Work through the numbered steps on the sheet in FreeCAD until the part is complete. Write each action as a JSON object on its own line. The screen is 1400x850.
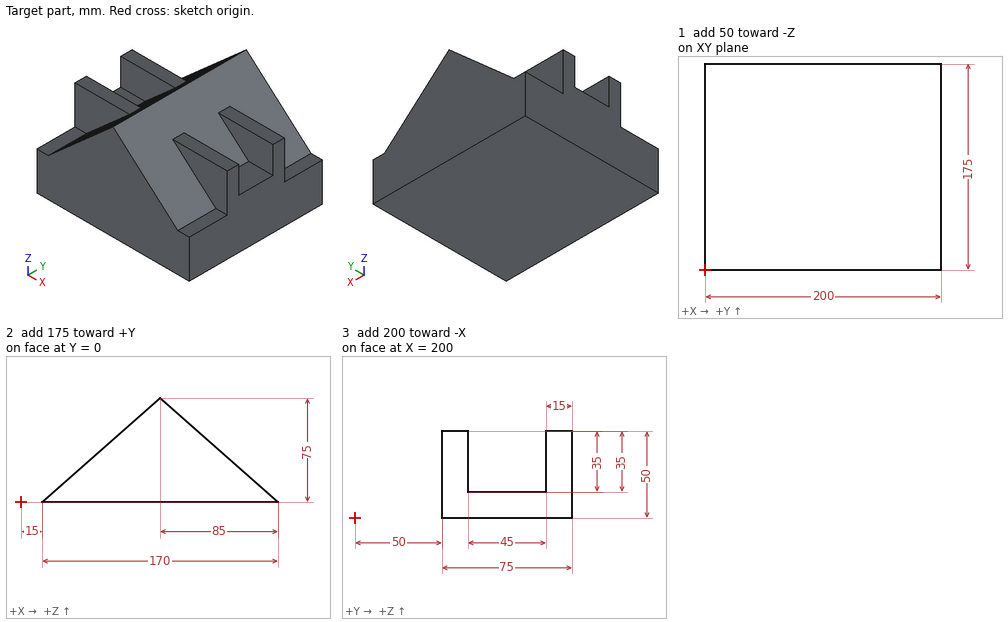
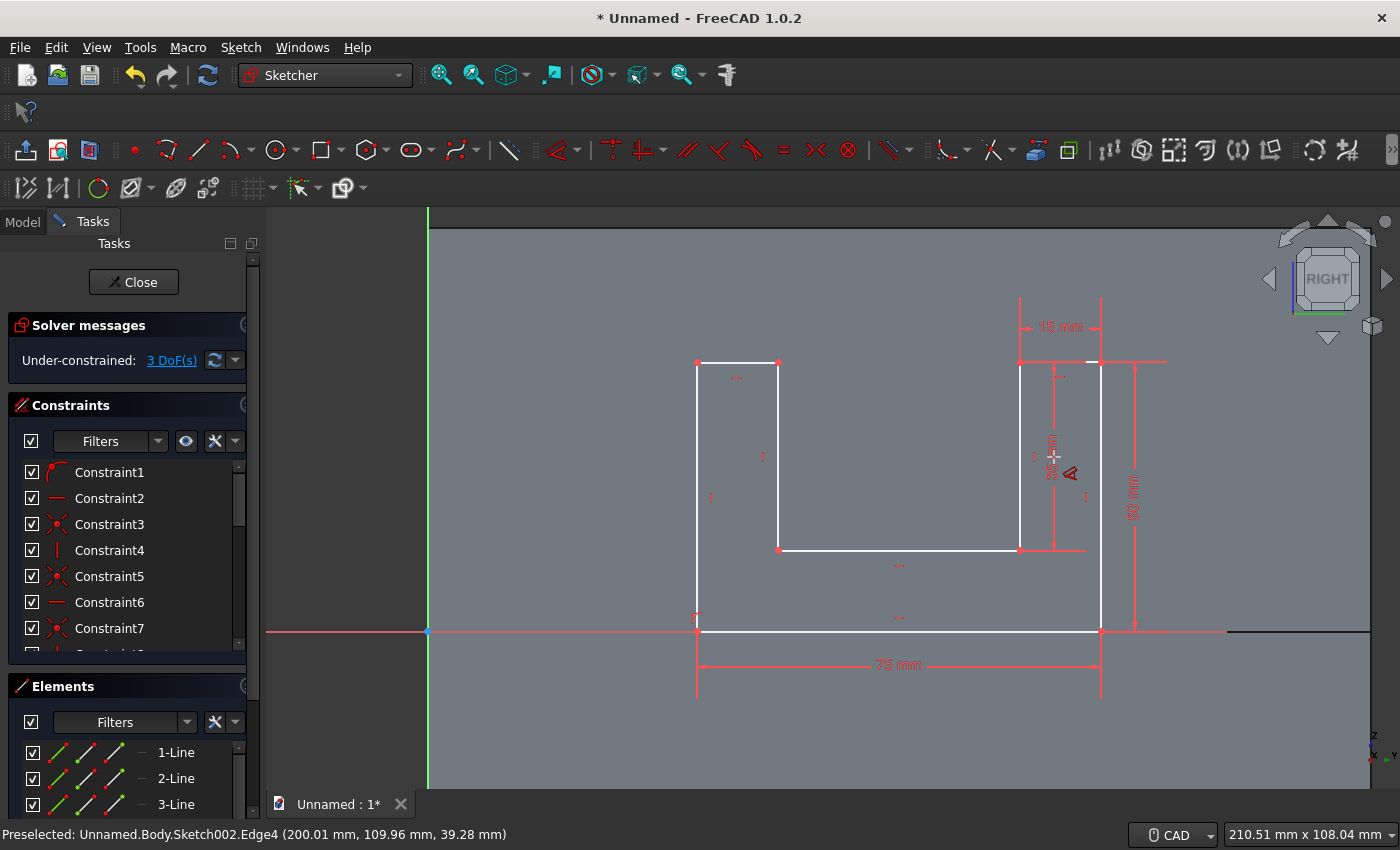
{"action": "left_click", "coordinate": [948, 551]}
{"action": "left_click", "coordinate": [899, 585]}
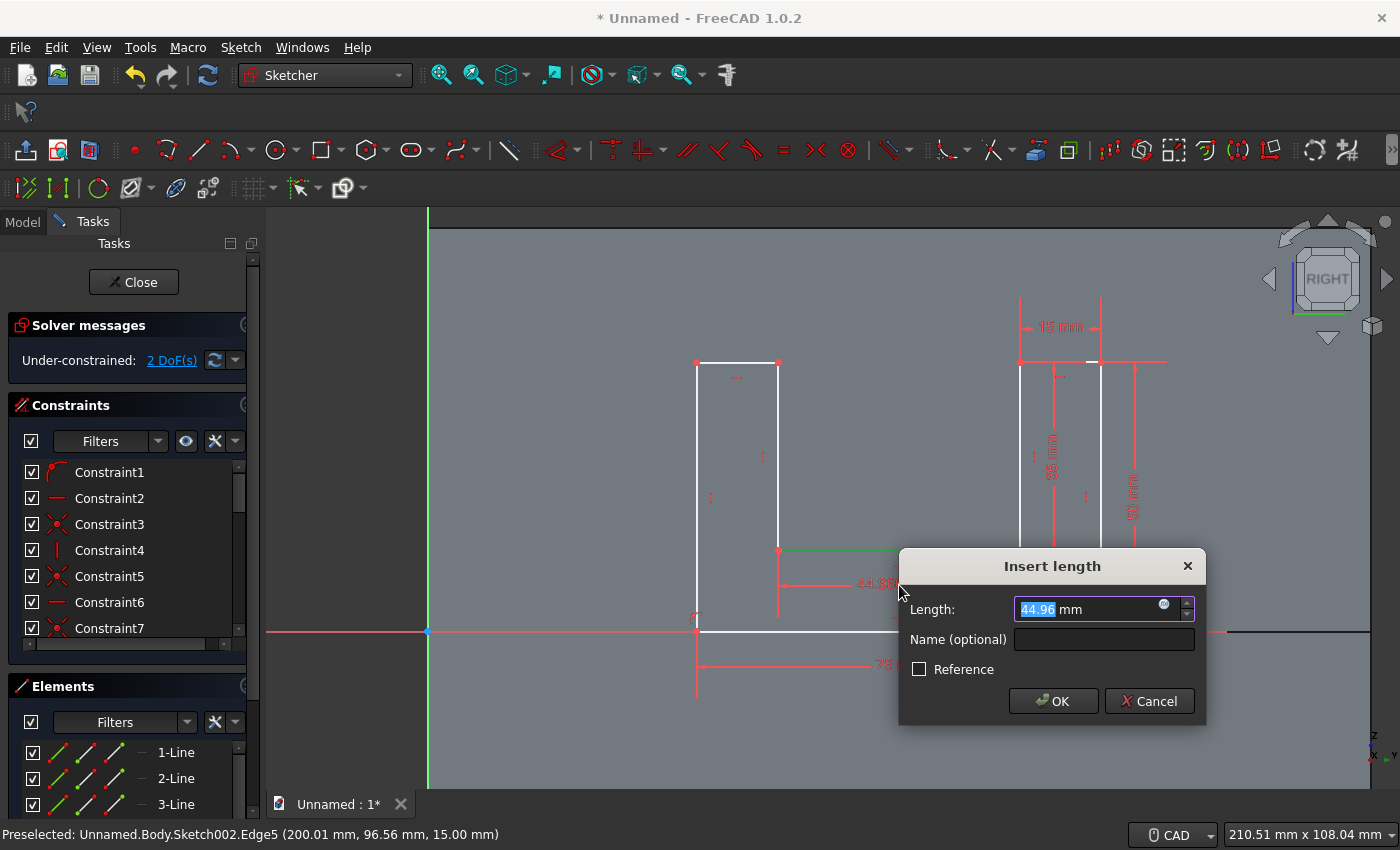
{"action": "type", "text": "45"}
{"action": "key", "text": "Return"}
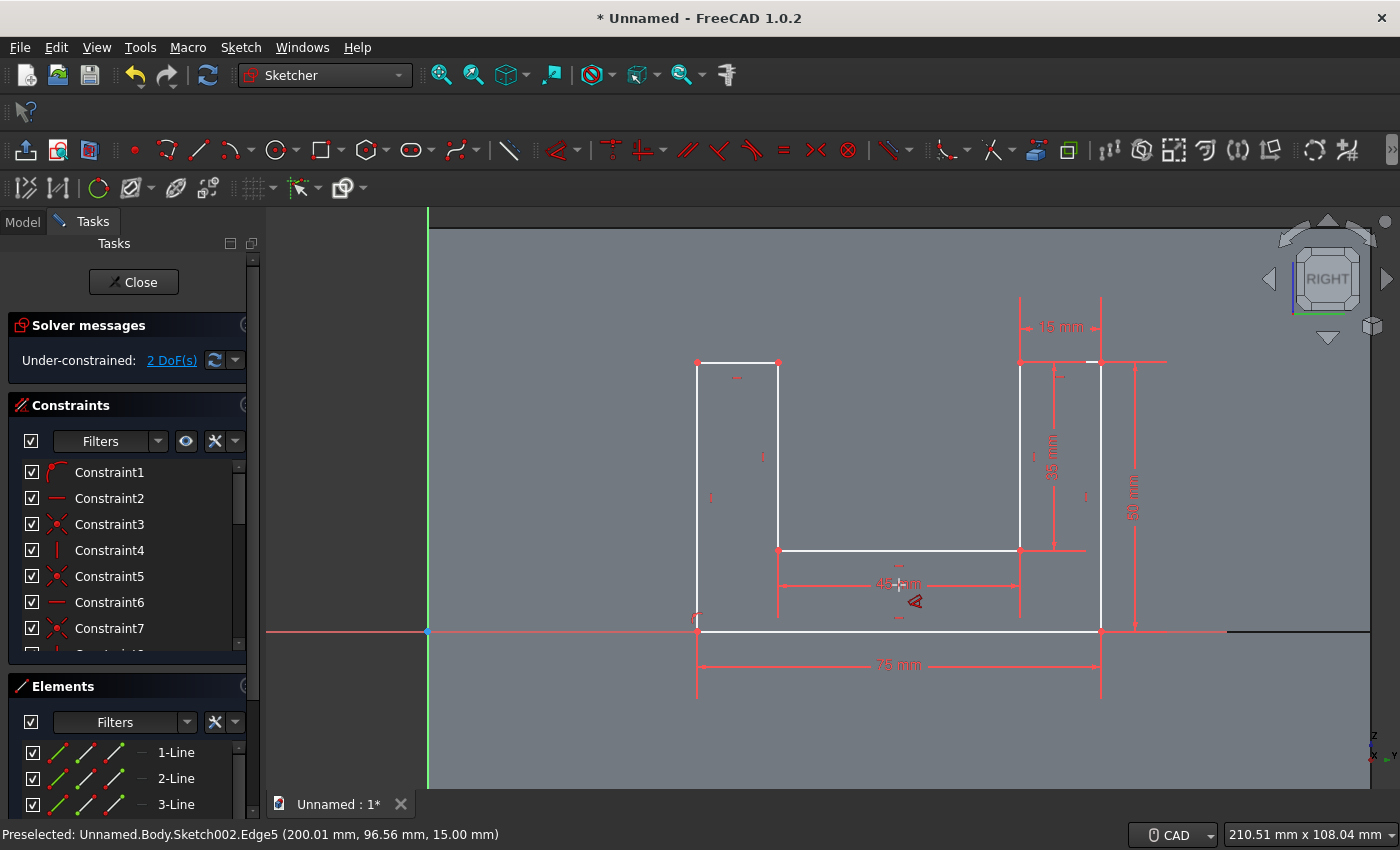
{"action": "left_click", "coordinate": [778, 494]}
{"action": "left_click", "coordinate": [812, 457]}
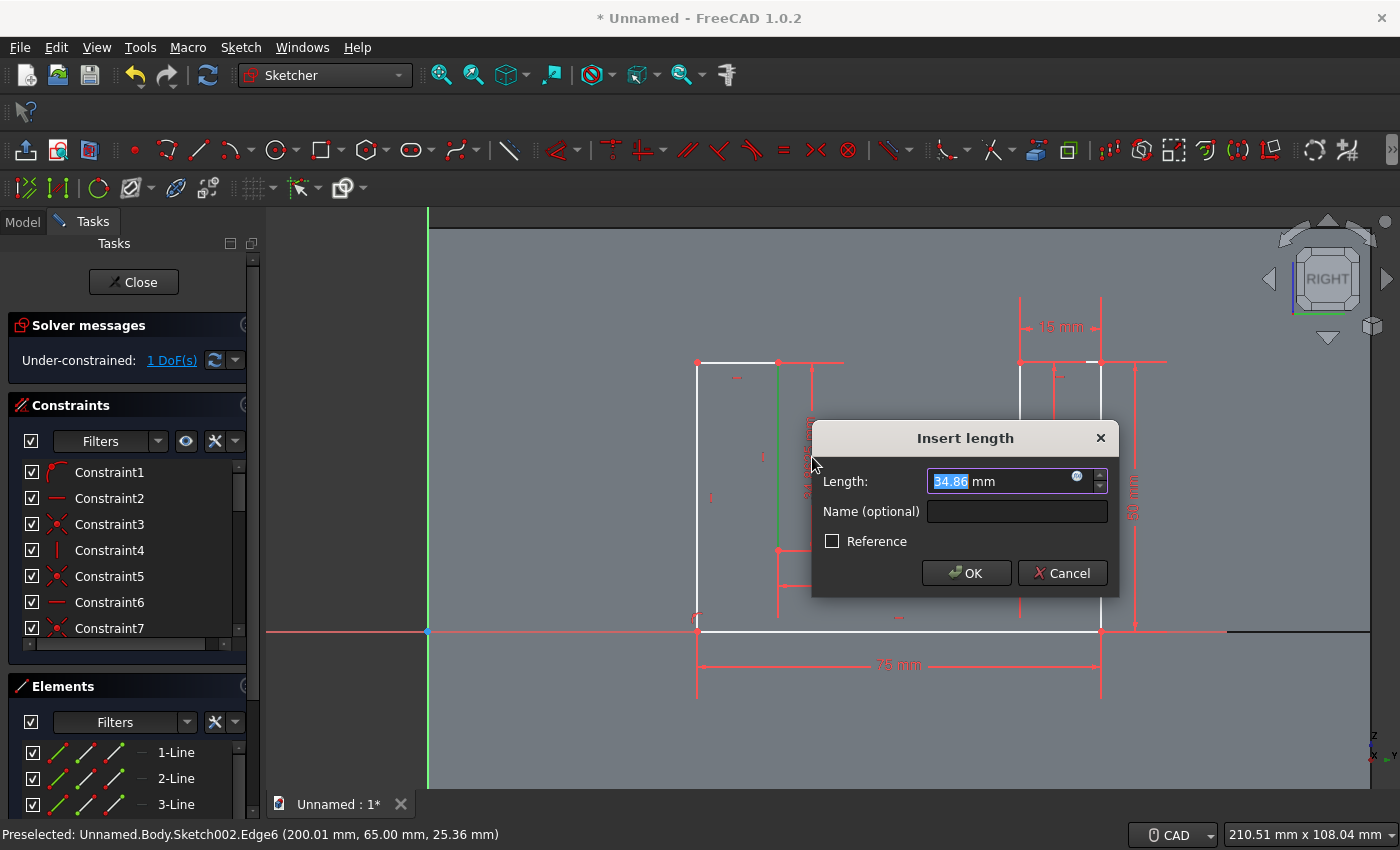
{"action": "type", "text": "35"}
{"action": "key", "text": "Return"}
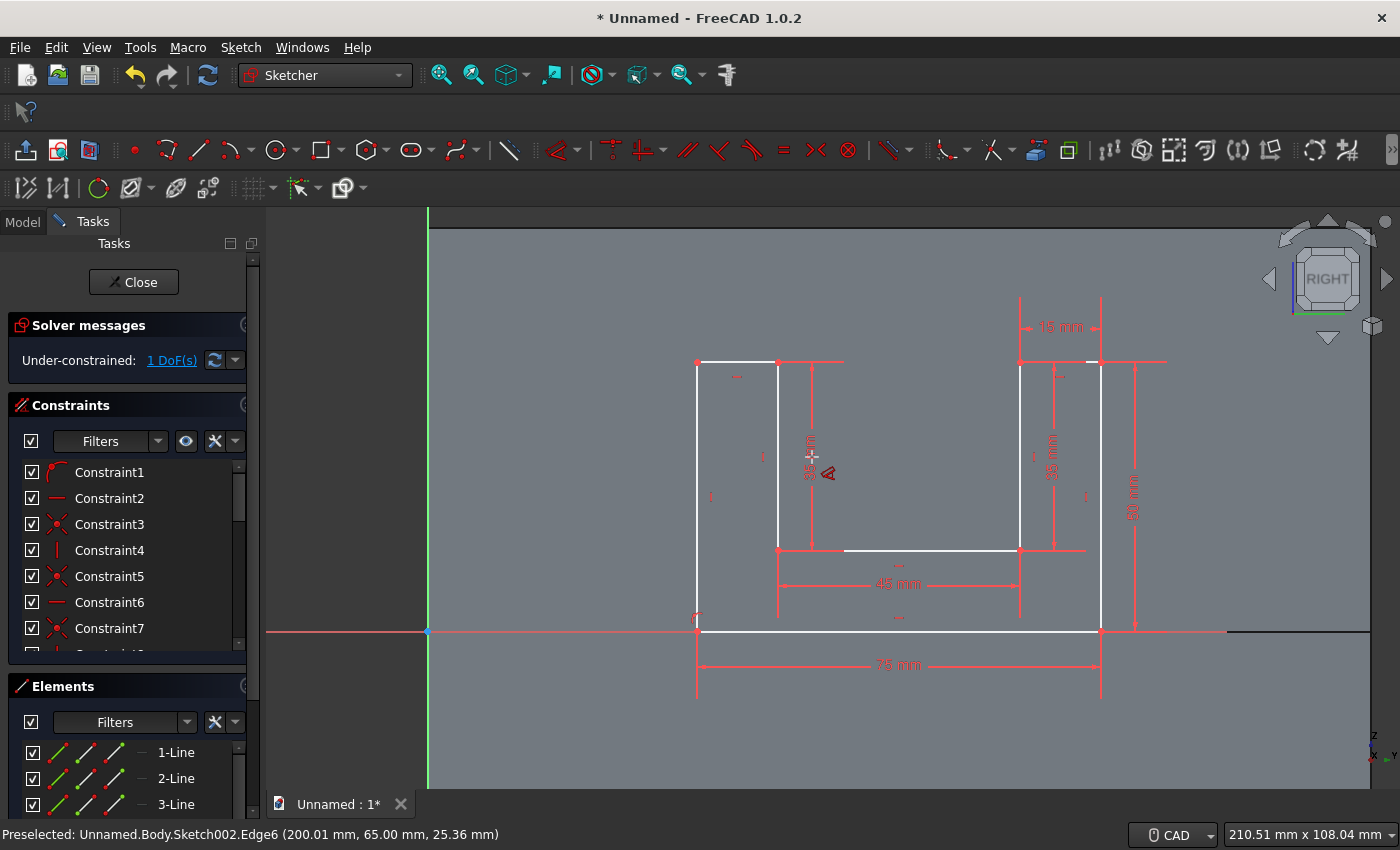
{"action": "left_click", "coordinate": [697, 632]}
{"action": "left_click", "coordinate": [563, 666]}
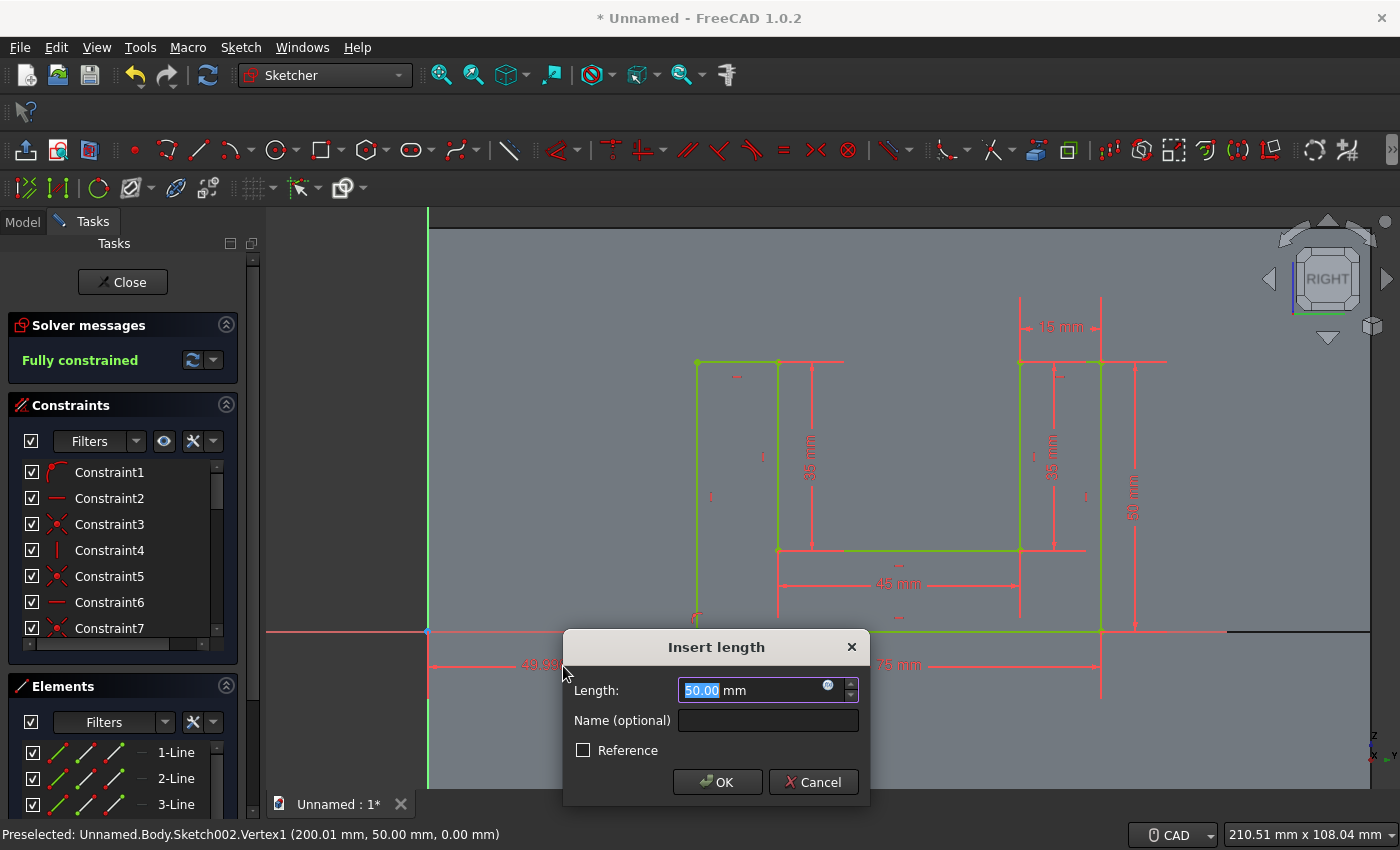
{"action": "type", "text": "50"}
{"action": "key", "text": "Return"}
{"action": "key", "text": "Escape"}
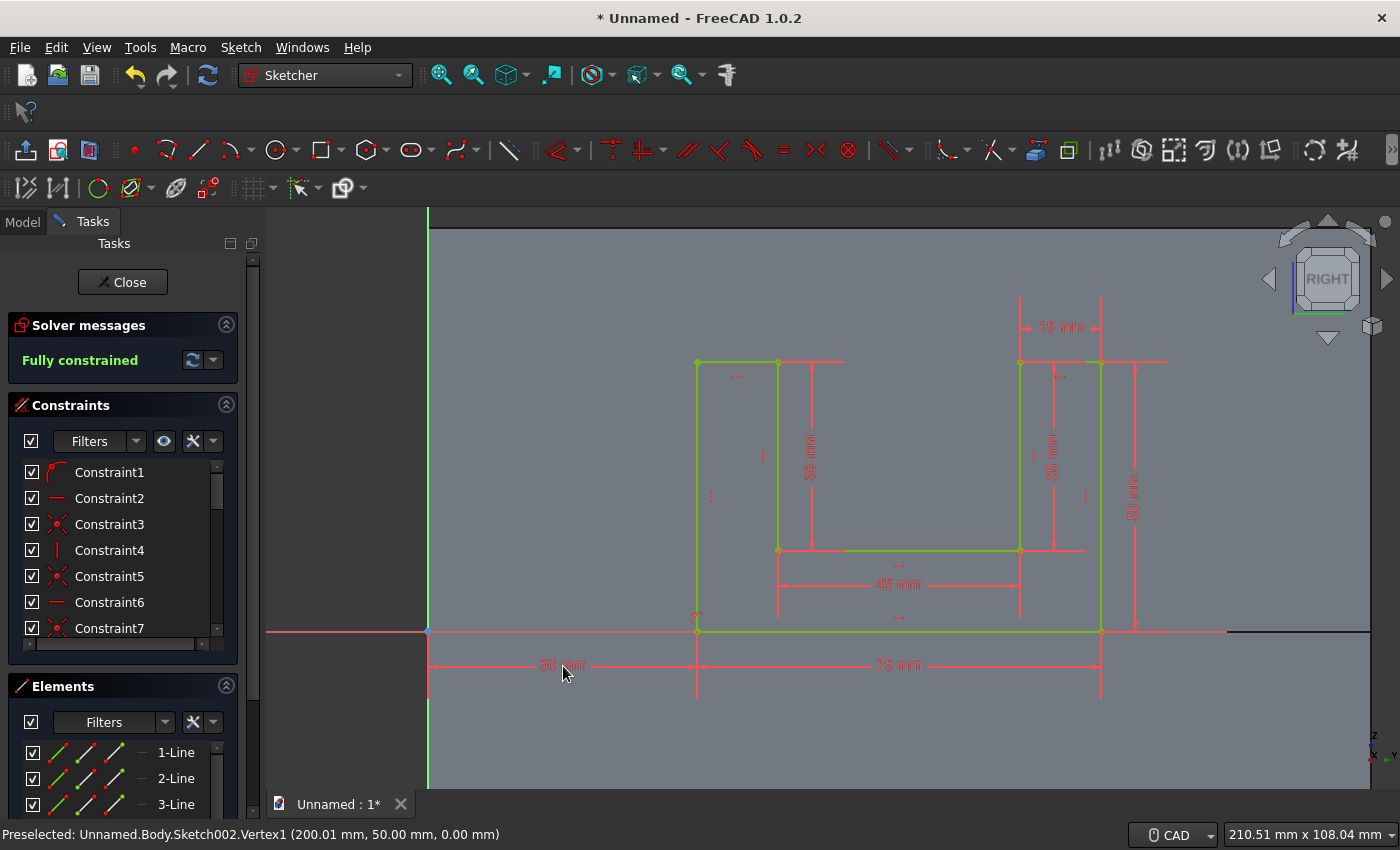
{"action": "left_click", "coordinate": [123, 282]}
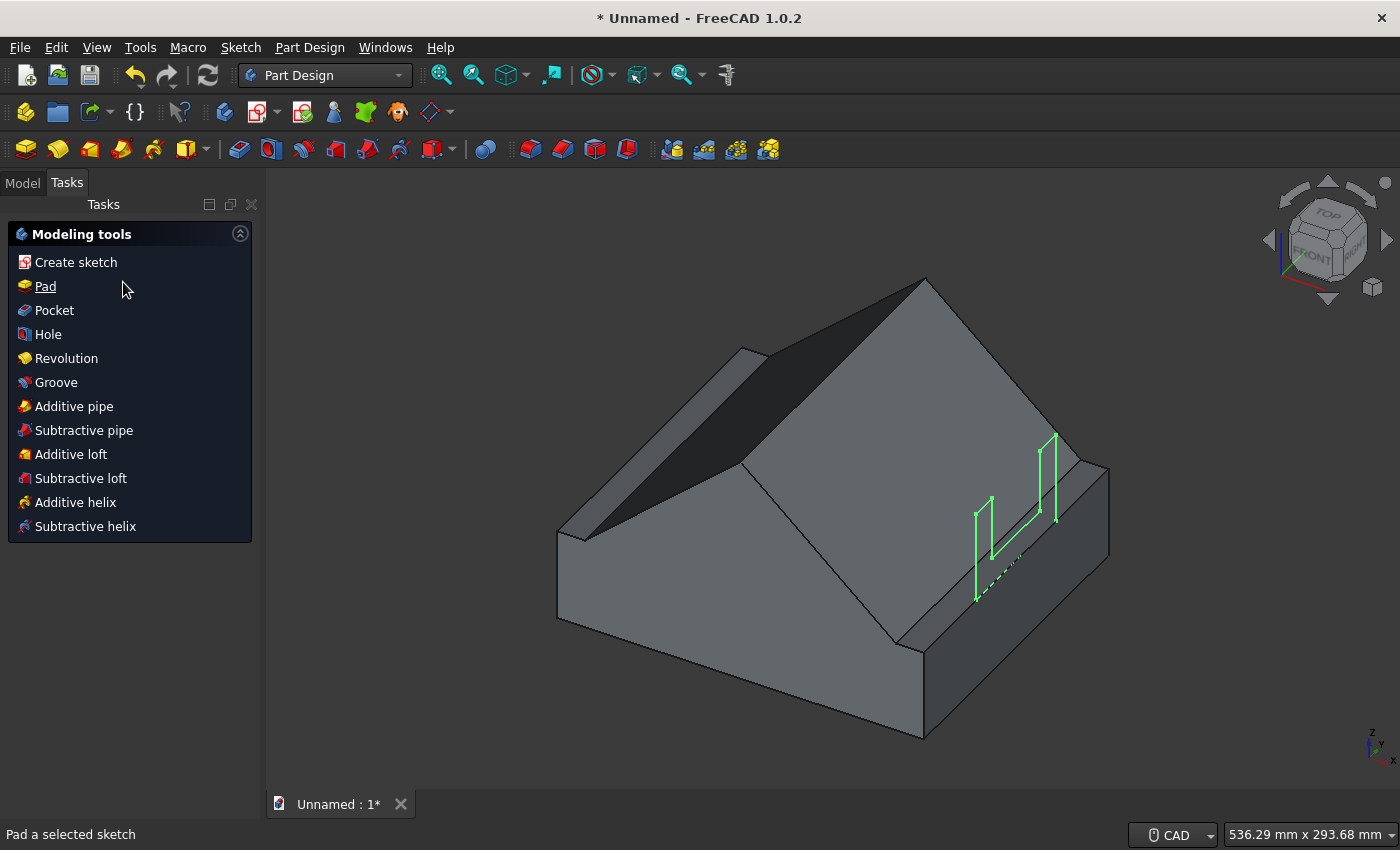
{"action": "left_click", "coordinate": [26, 150]}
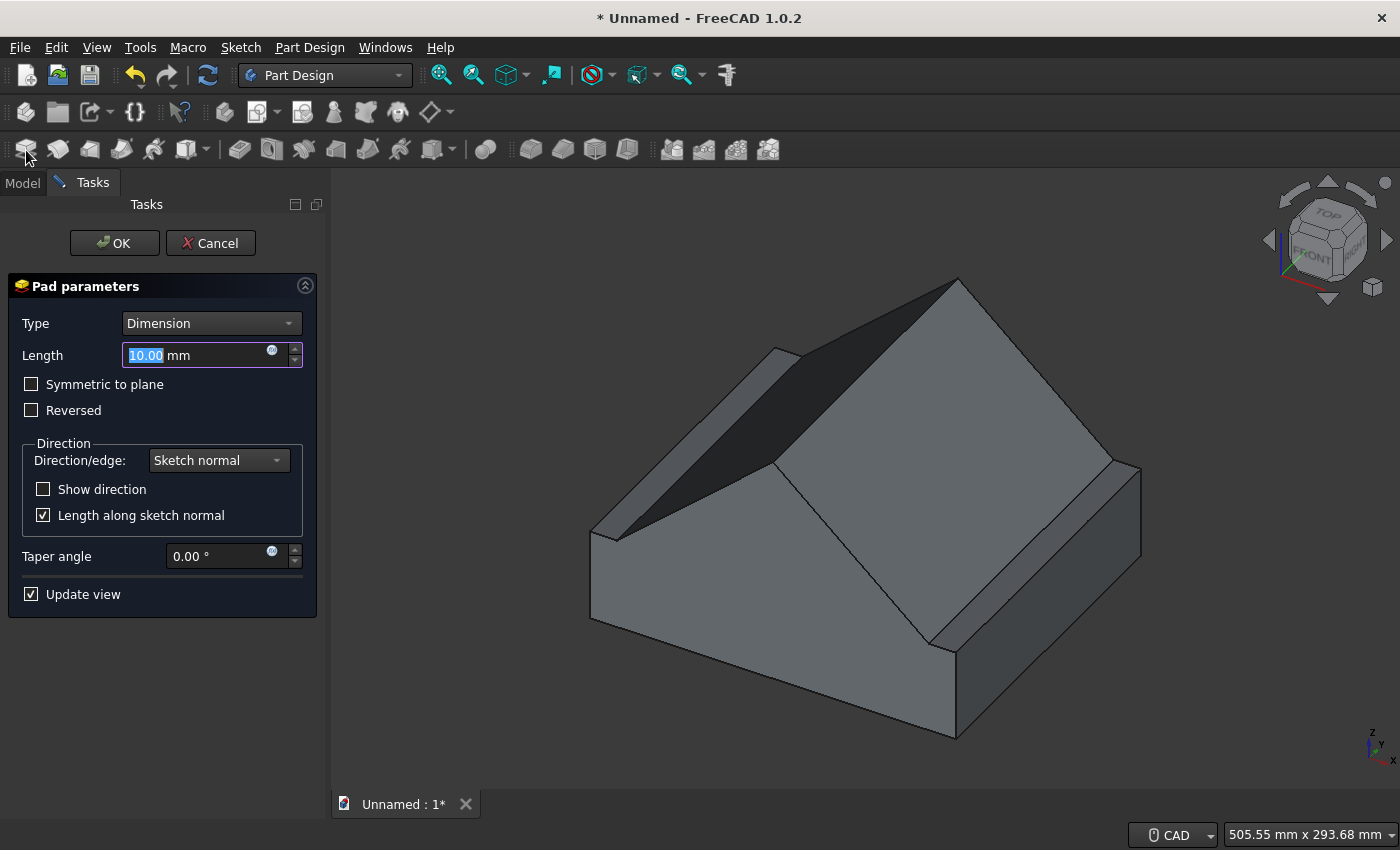
{"action": "type", "text": "200"}
{"action": "key", "text": "Tab"}